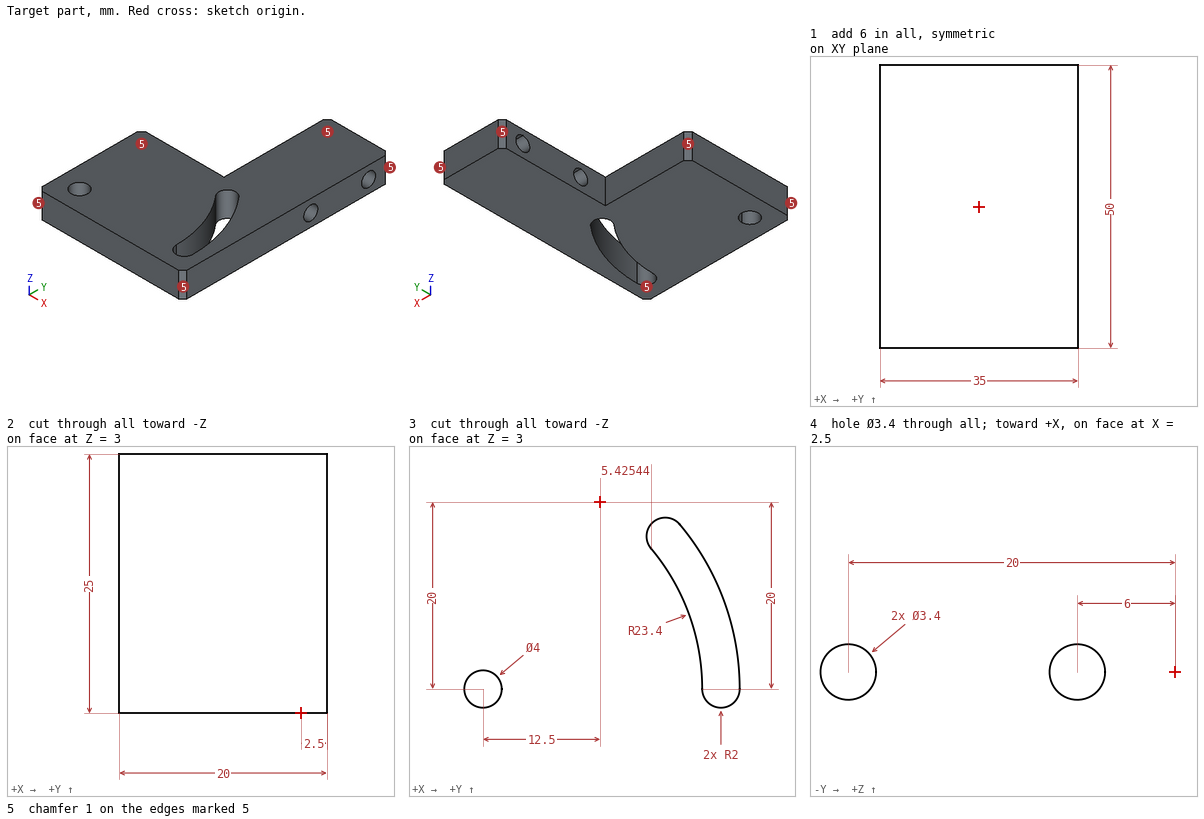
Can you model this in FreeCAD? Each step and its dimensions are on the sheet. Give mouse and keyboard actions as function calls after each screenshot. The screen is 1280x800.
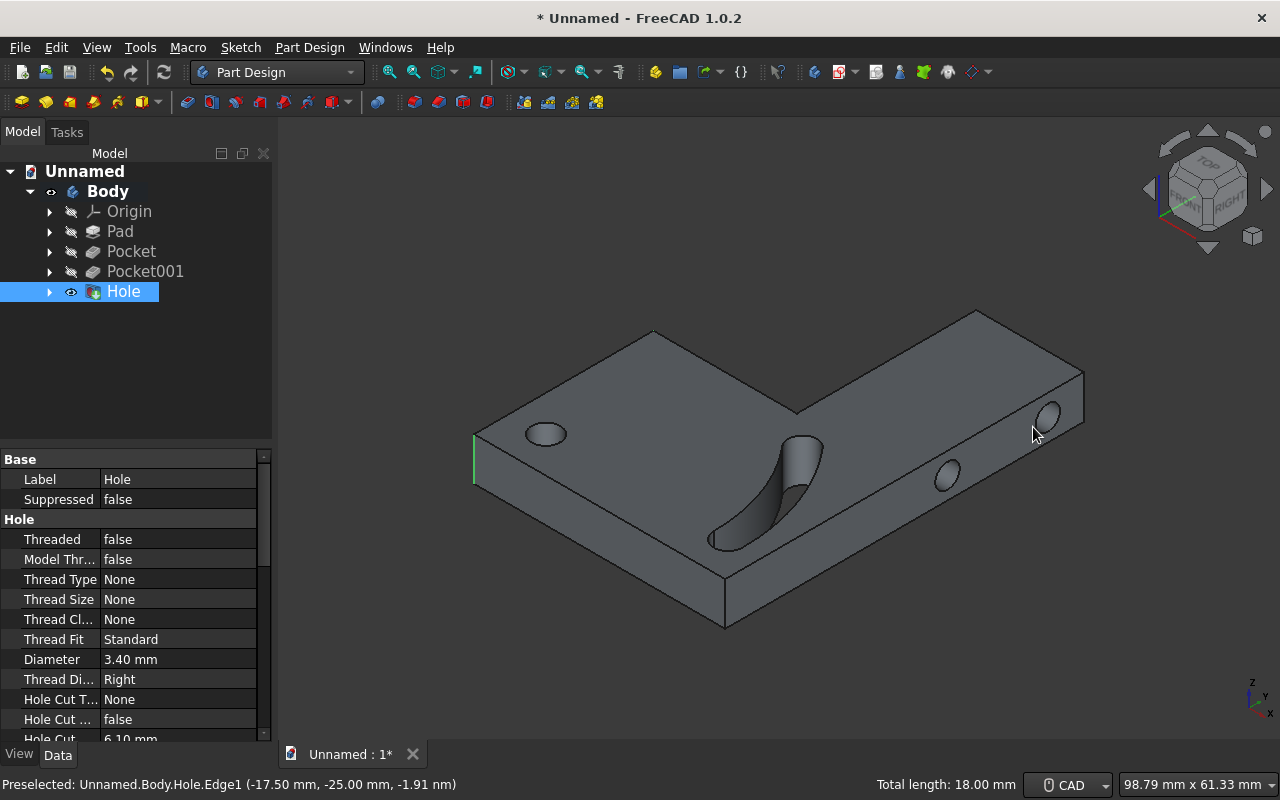
click(725, 603, ctrl)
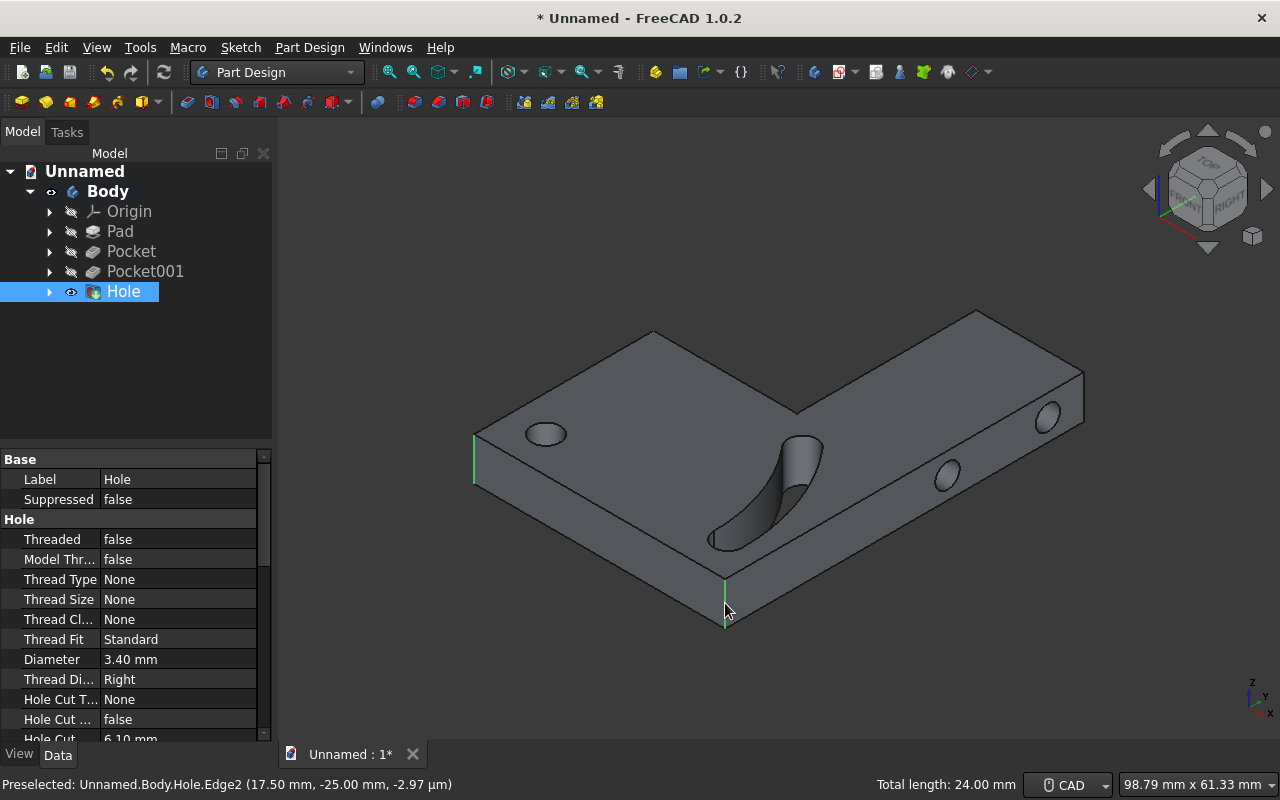
key(2)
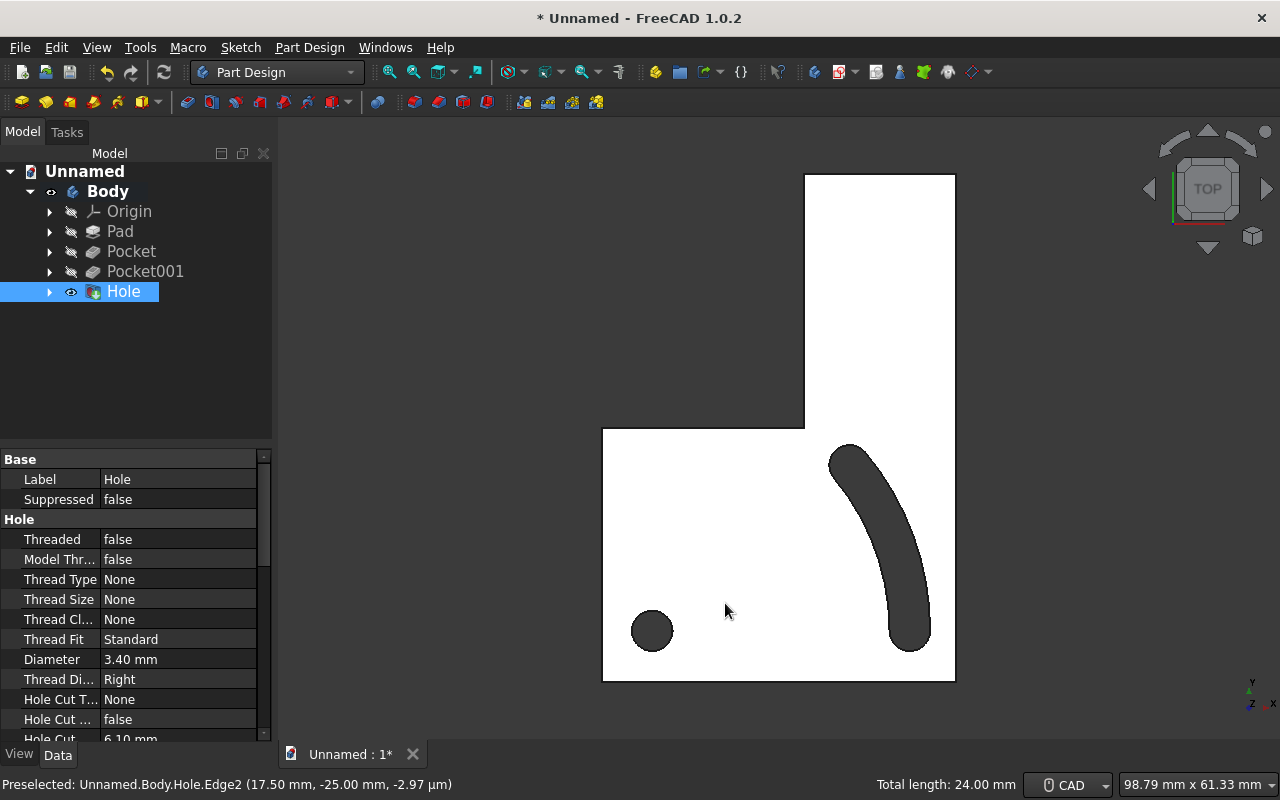
key(1)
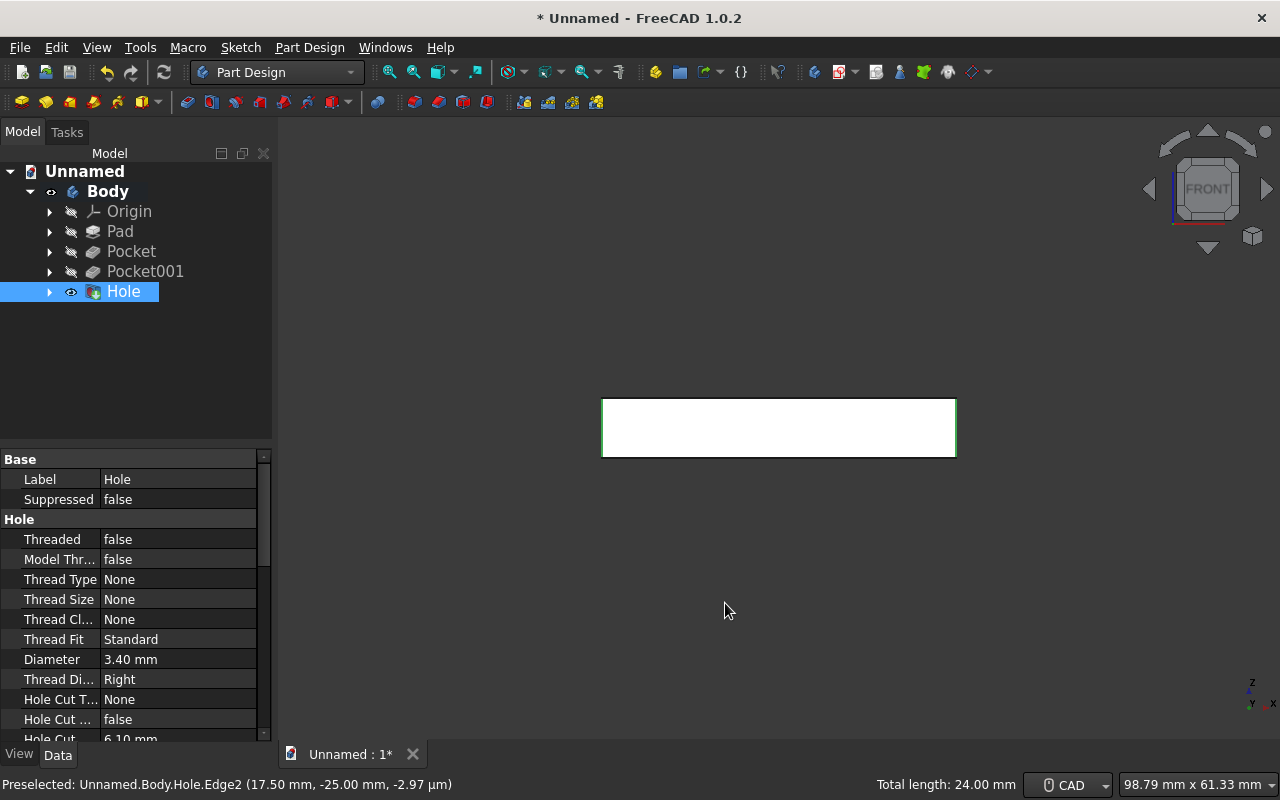
key(v)
key(f)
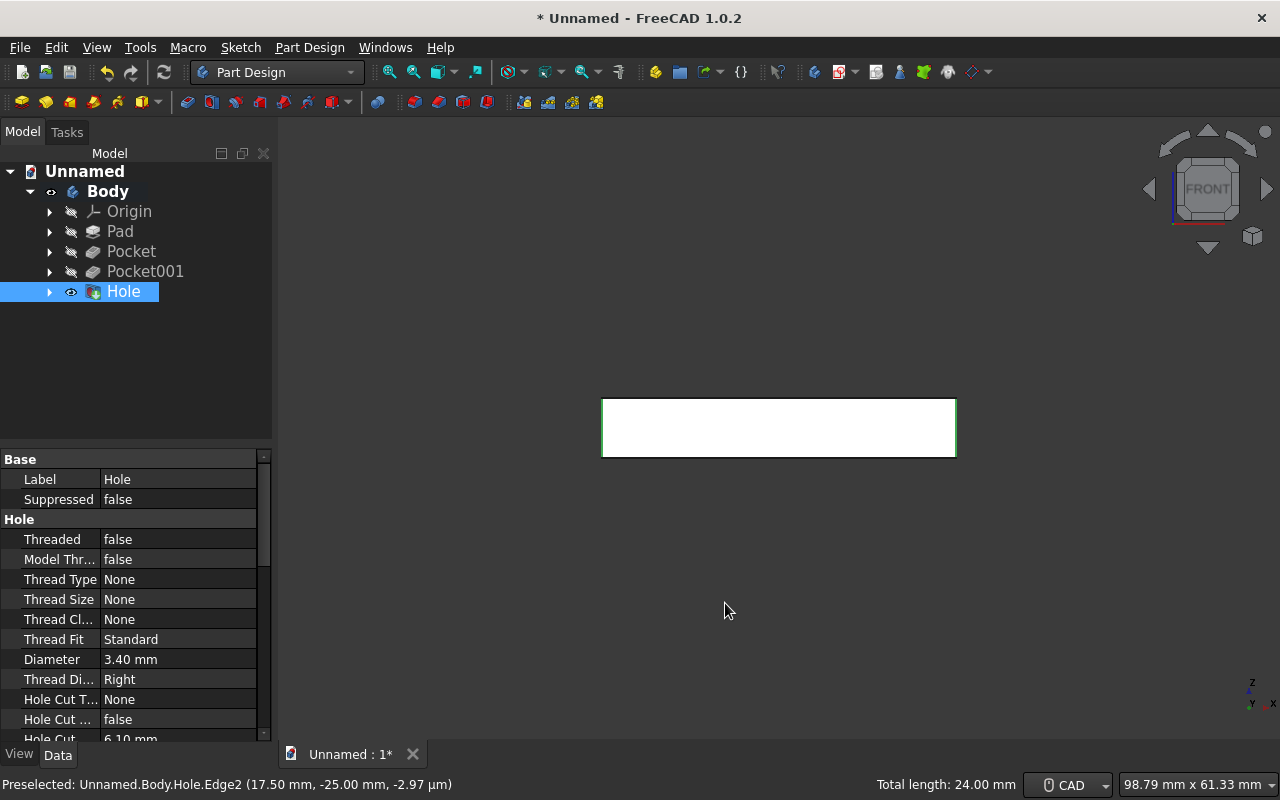
key(3)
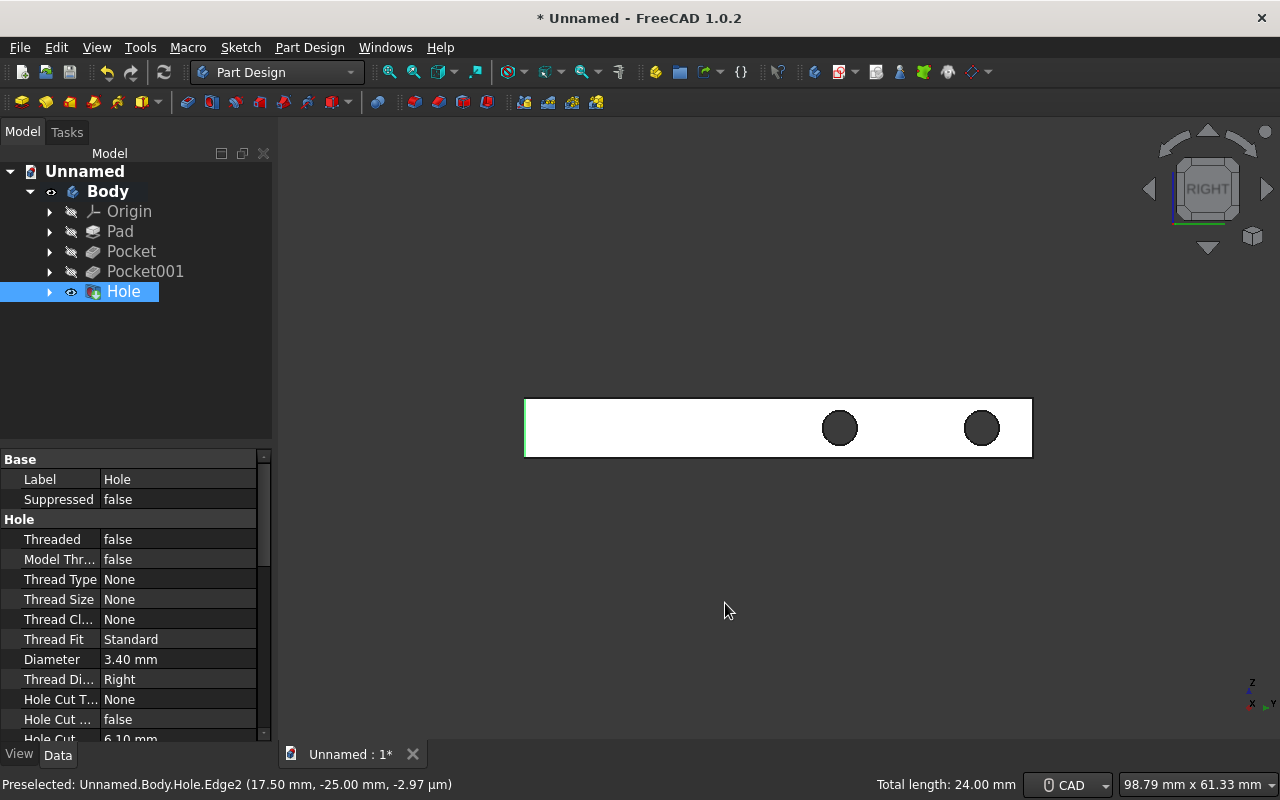
click(1033, 427, ctrl)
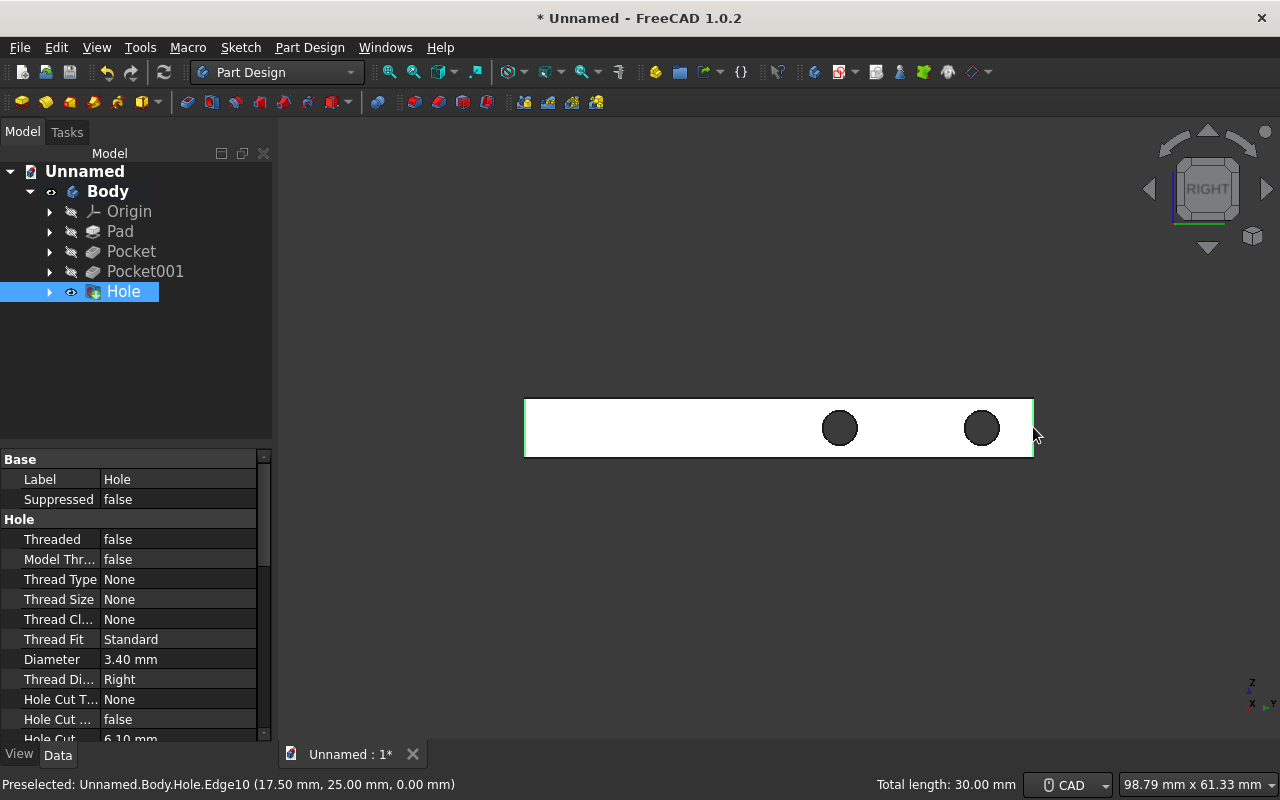
click(440, 102)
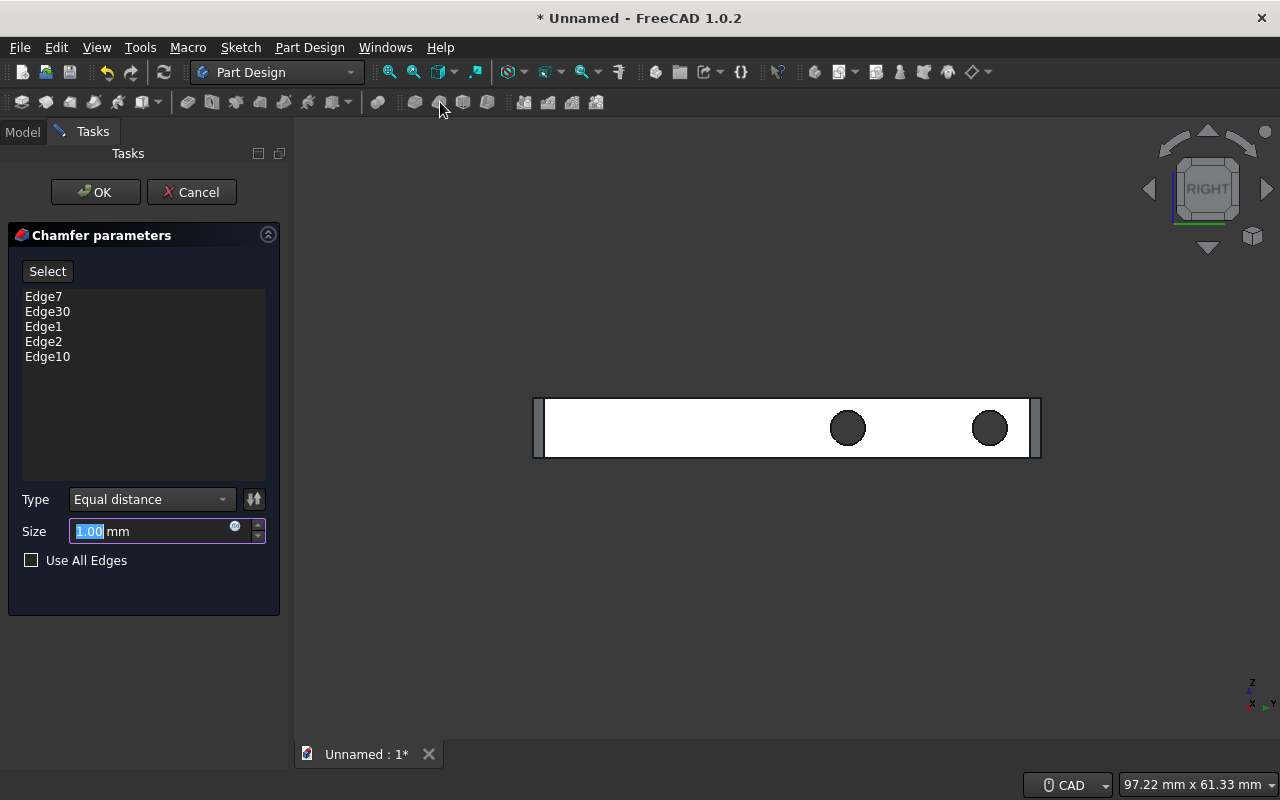
text(1)
key(Tab)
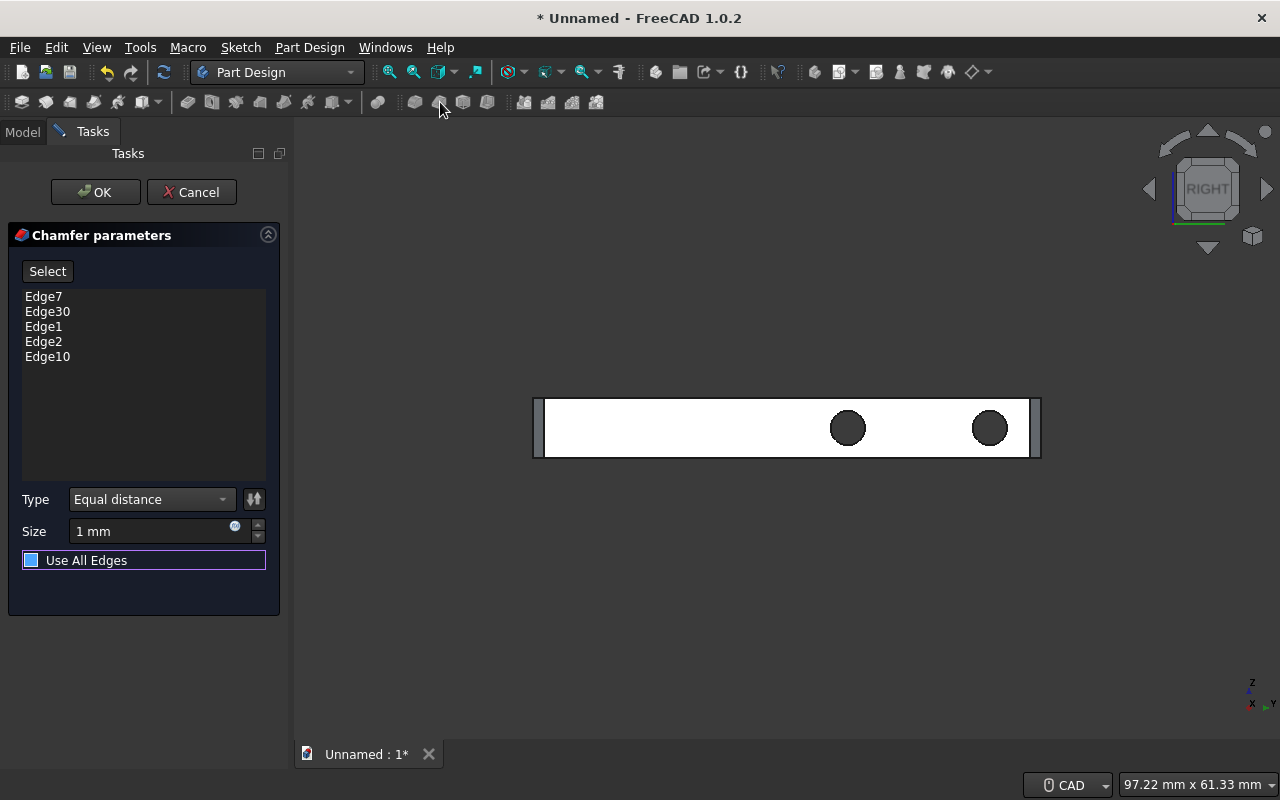
click(96, 192)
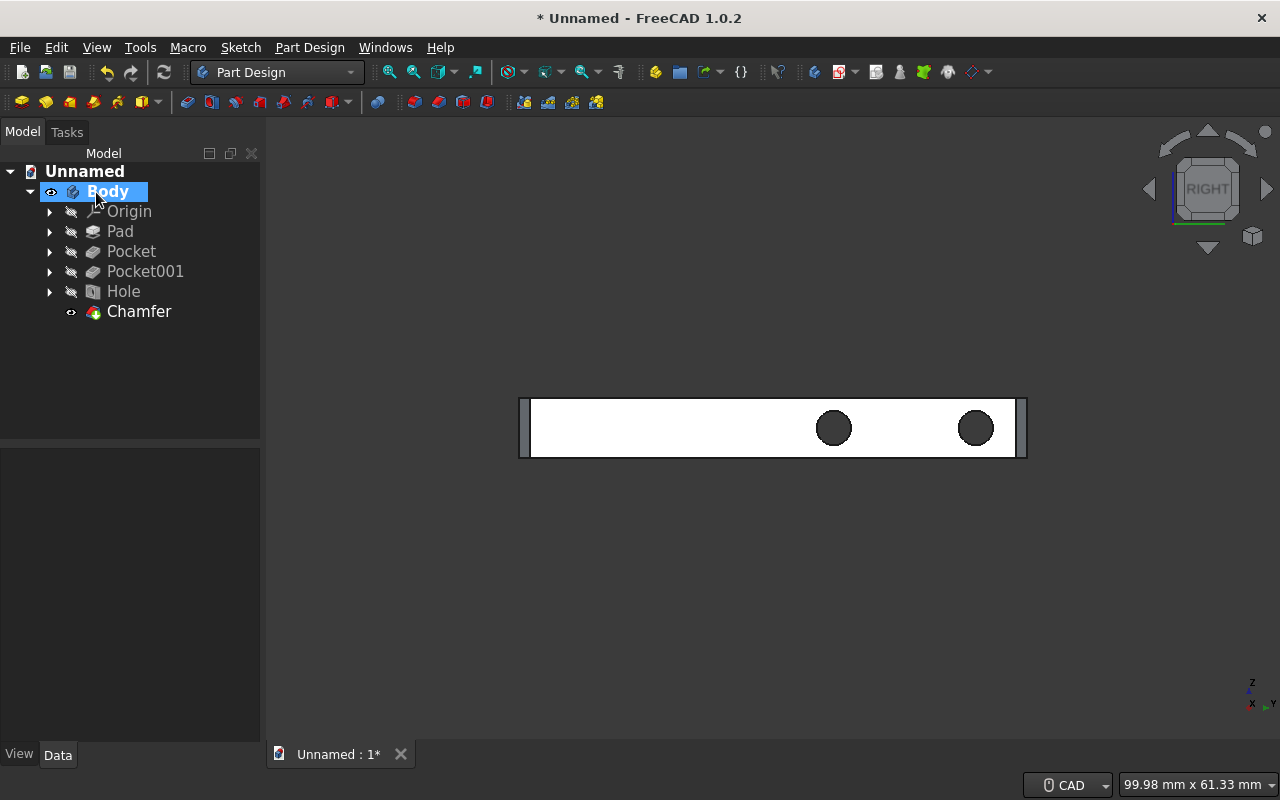
key(0)